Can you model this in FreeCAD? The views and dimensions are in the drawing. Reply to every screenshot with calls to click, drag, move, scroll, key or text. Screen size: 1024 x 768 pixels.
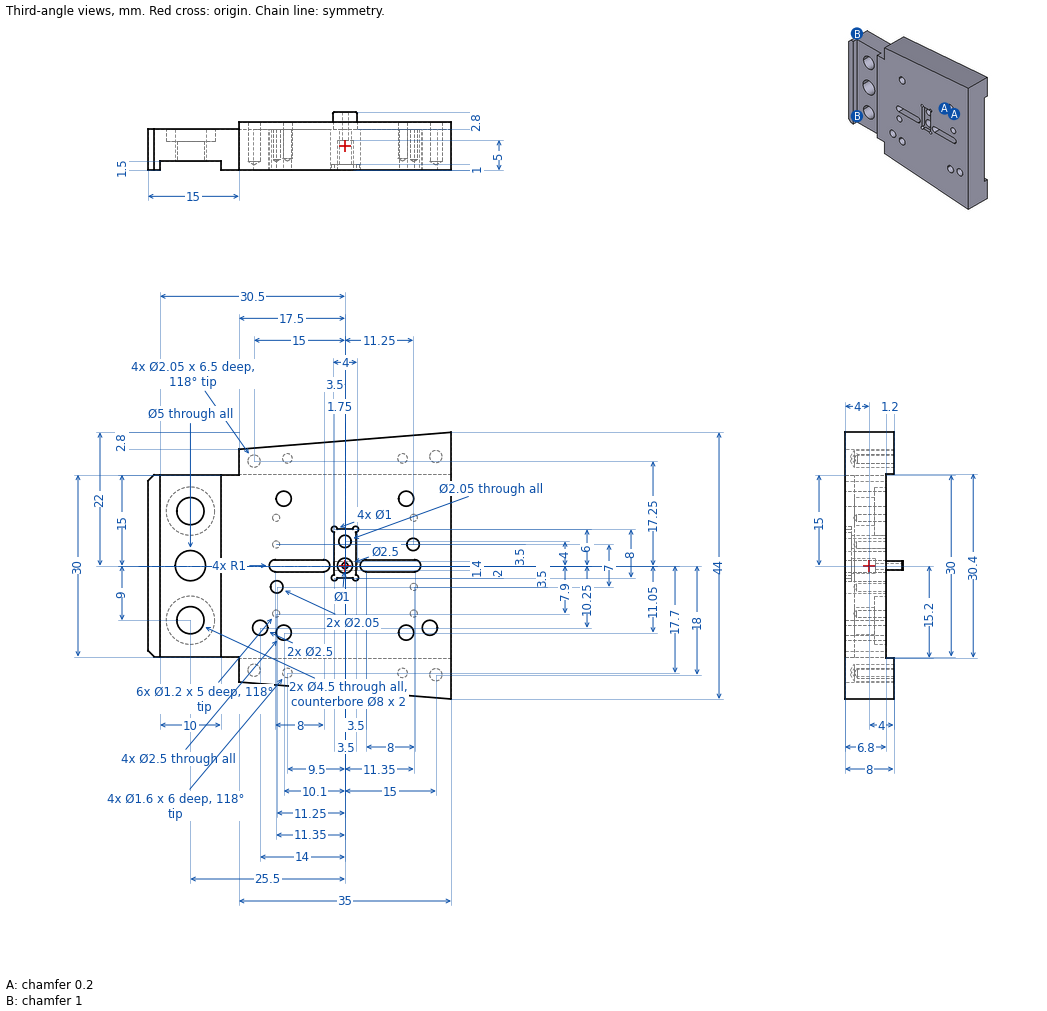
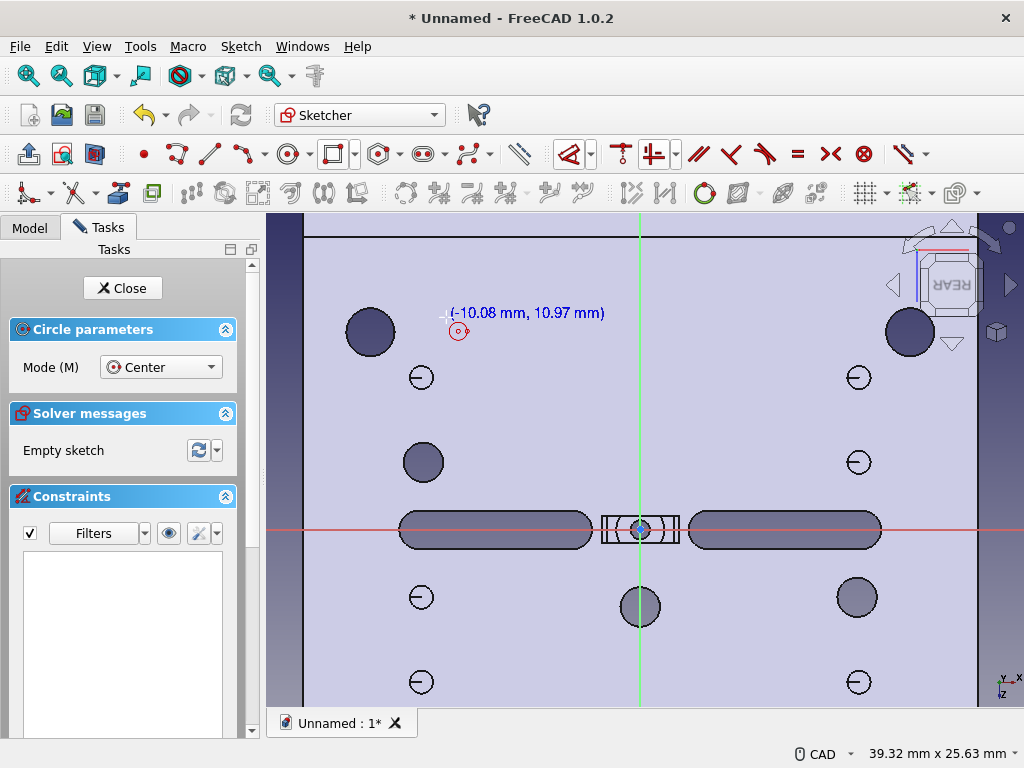
click(446, 317)
move(463, 300)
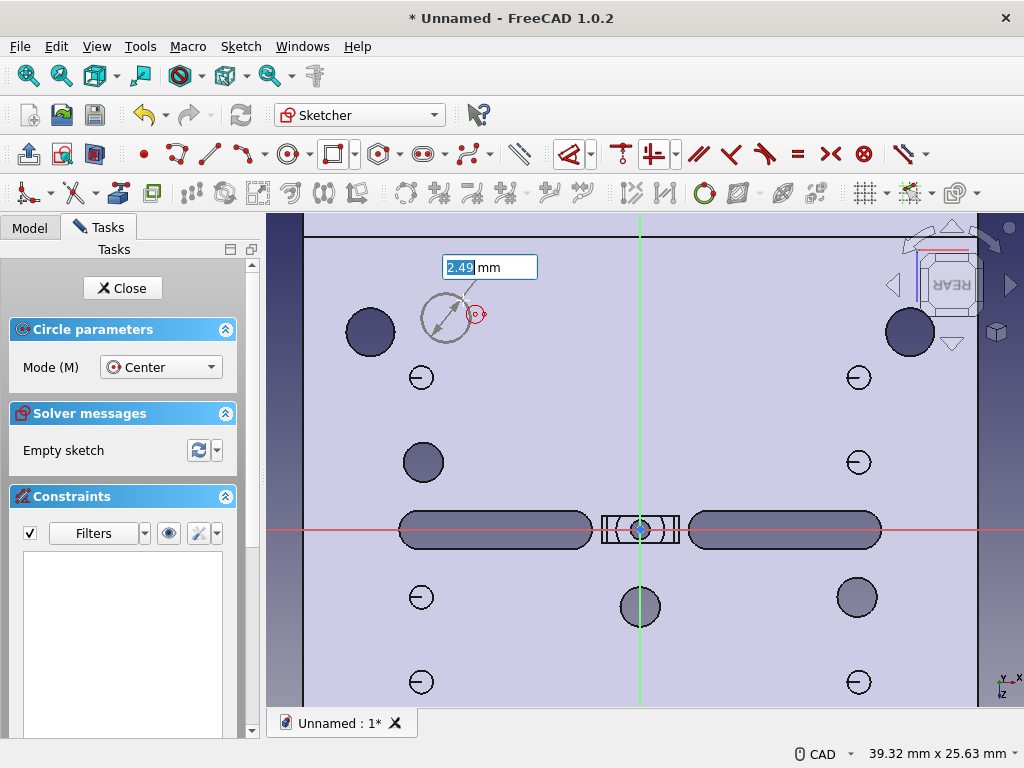
text(2.5)
key(Return)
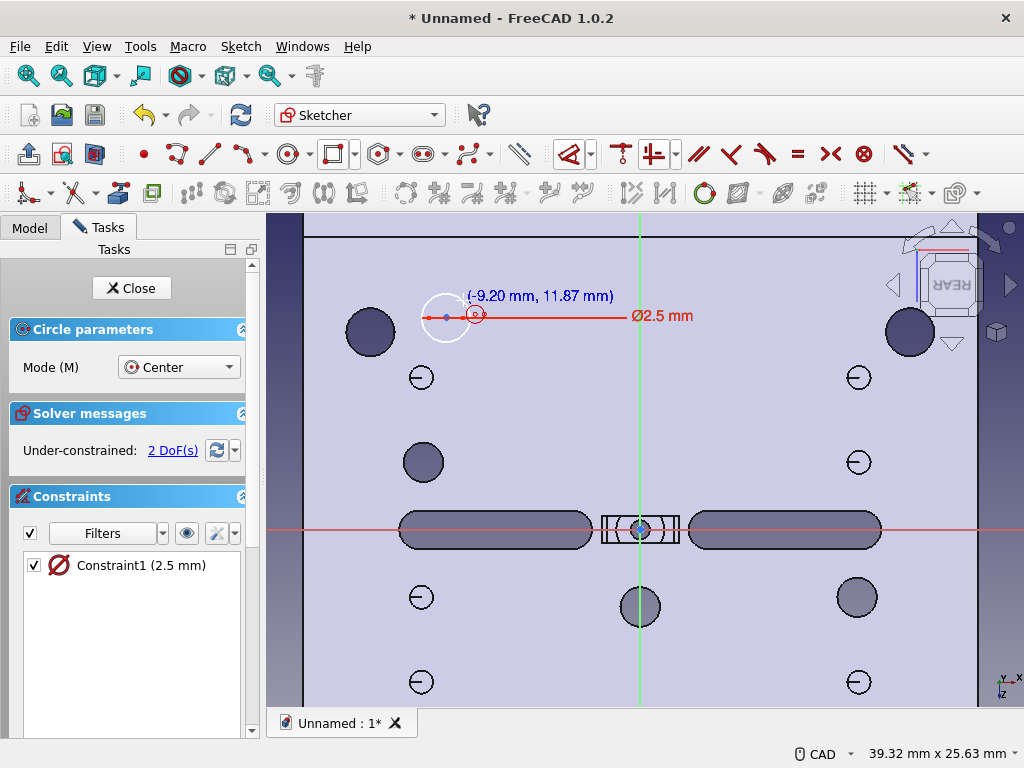
click(835, 317)
move(852, 300)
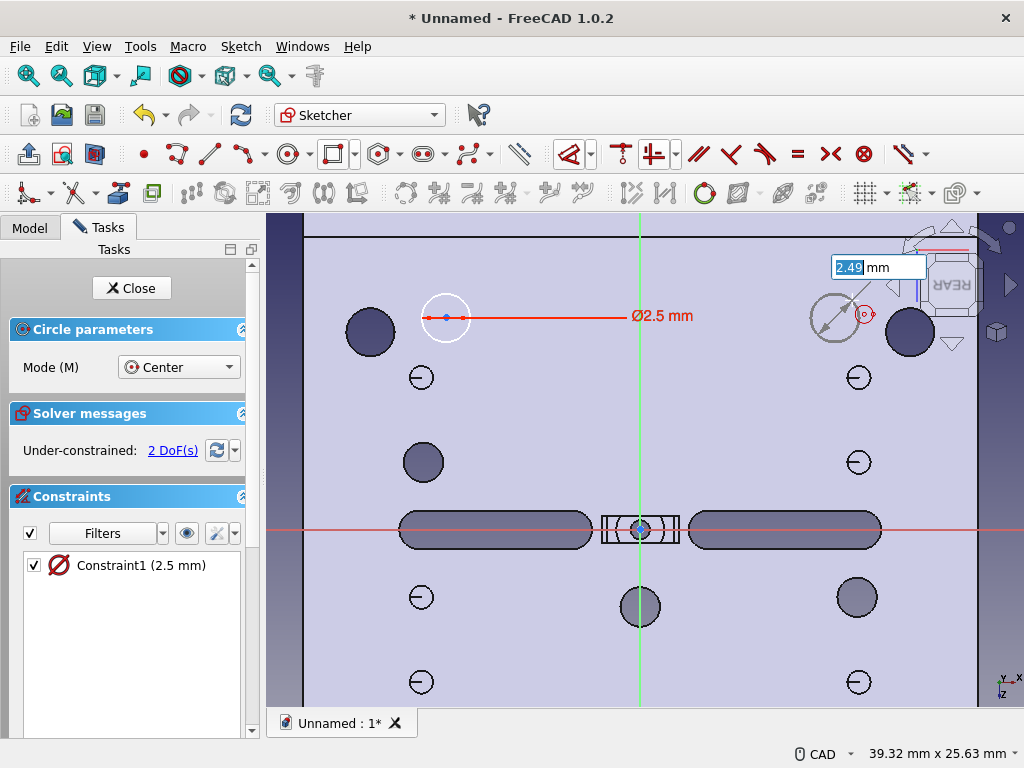
text(2.5)
key(Return)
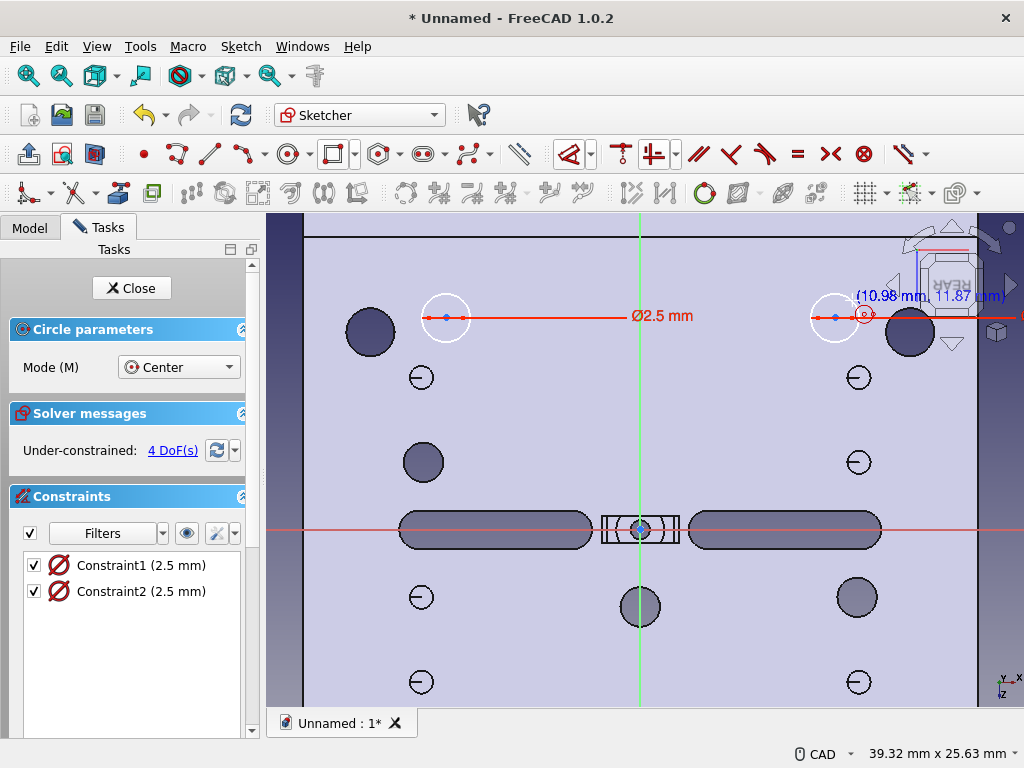
scroll(447, 318, down, 2)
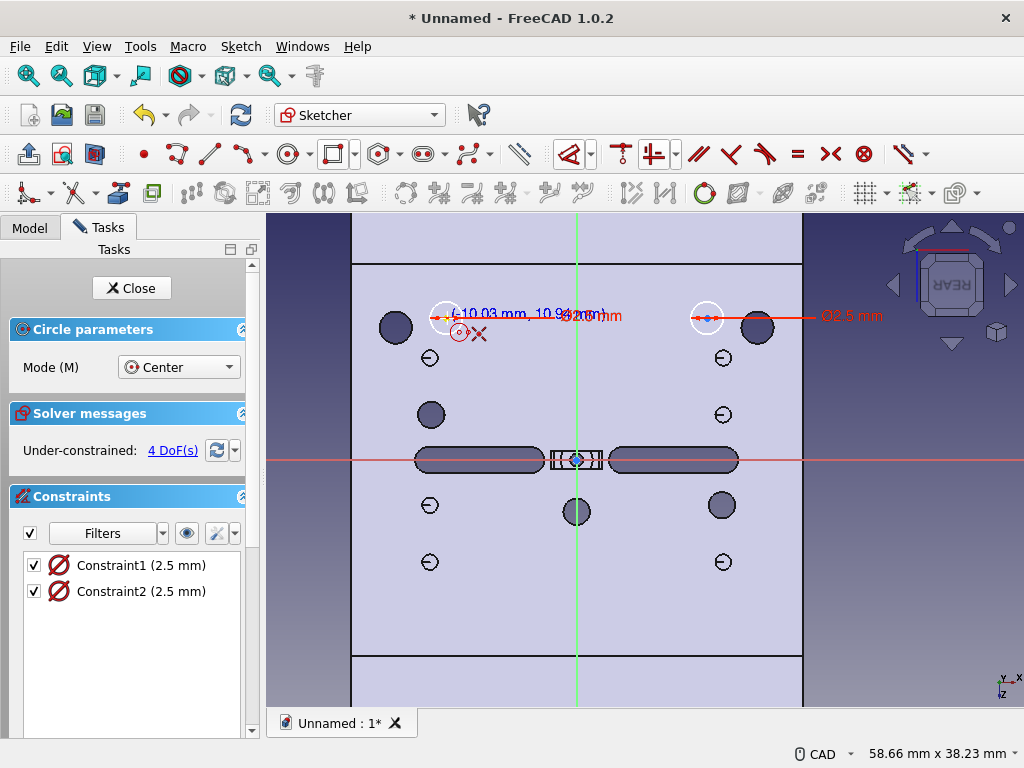
scroll(446, 603, up, 2)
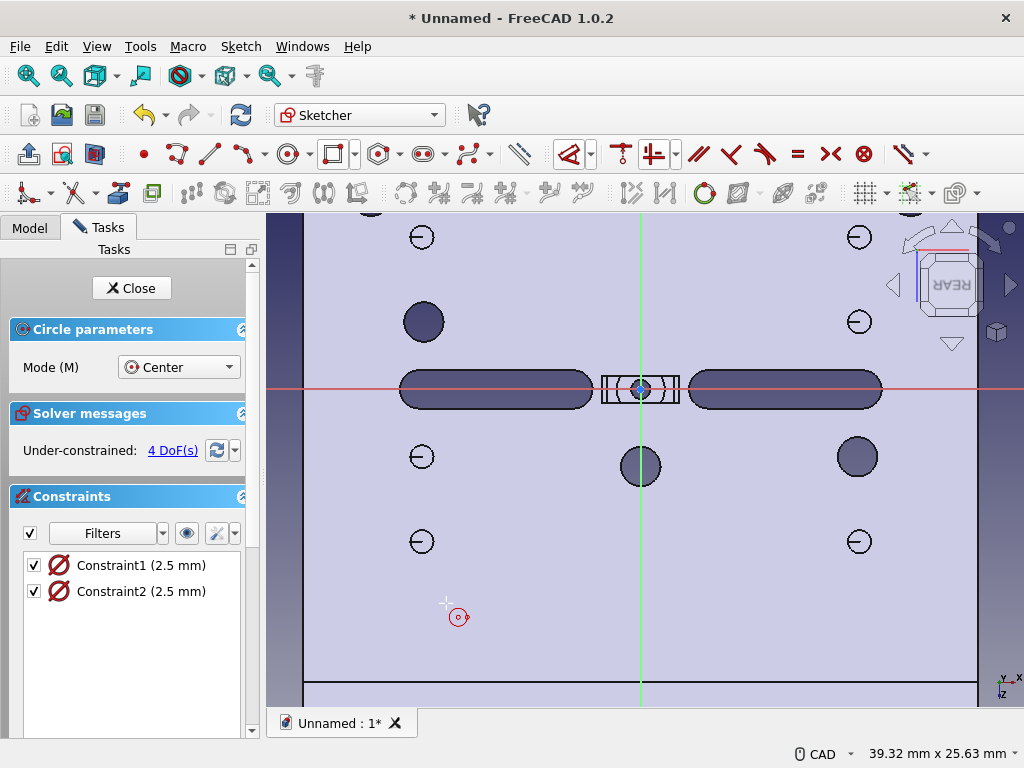
click(446, 602)
move(463, 585)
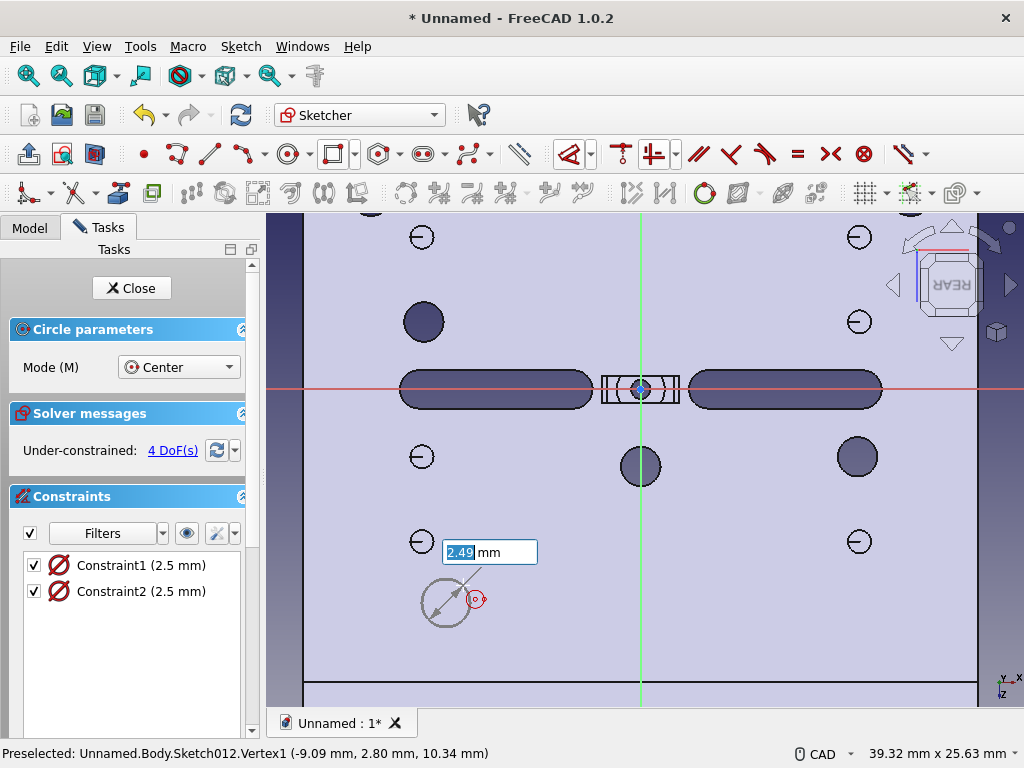
text(2.5)
key(Return)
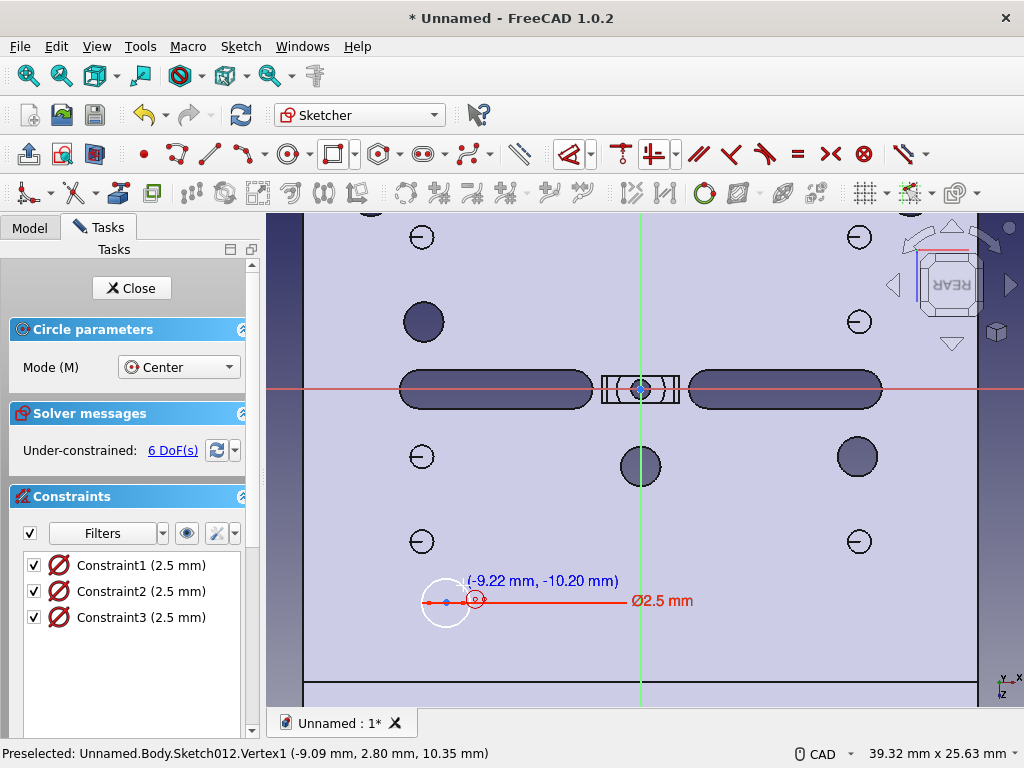
click(835, 602)
move(852, 585)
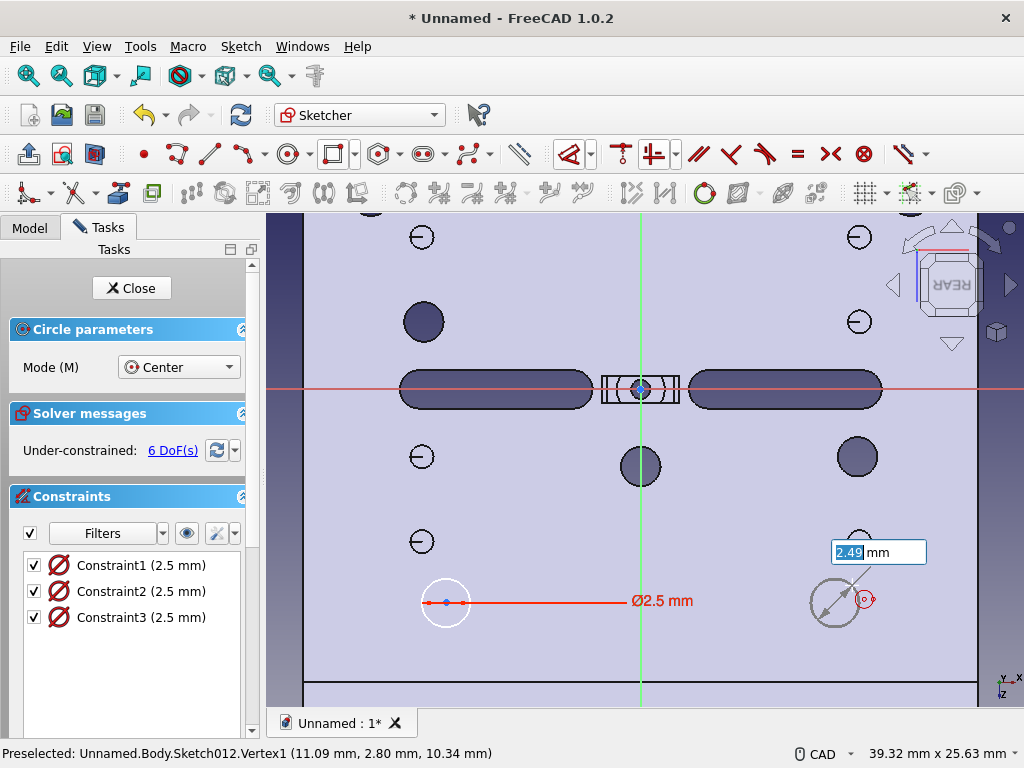
text(2.5)
key(Return)
key(Escape)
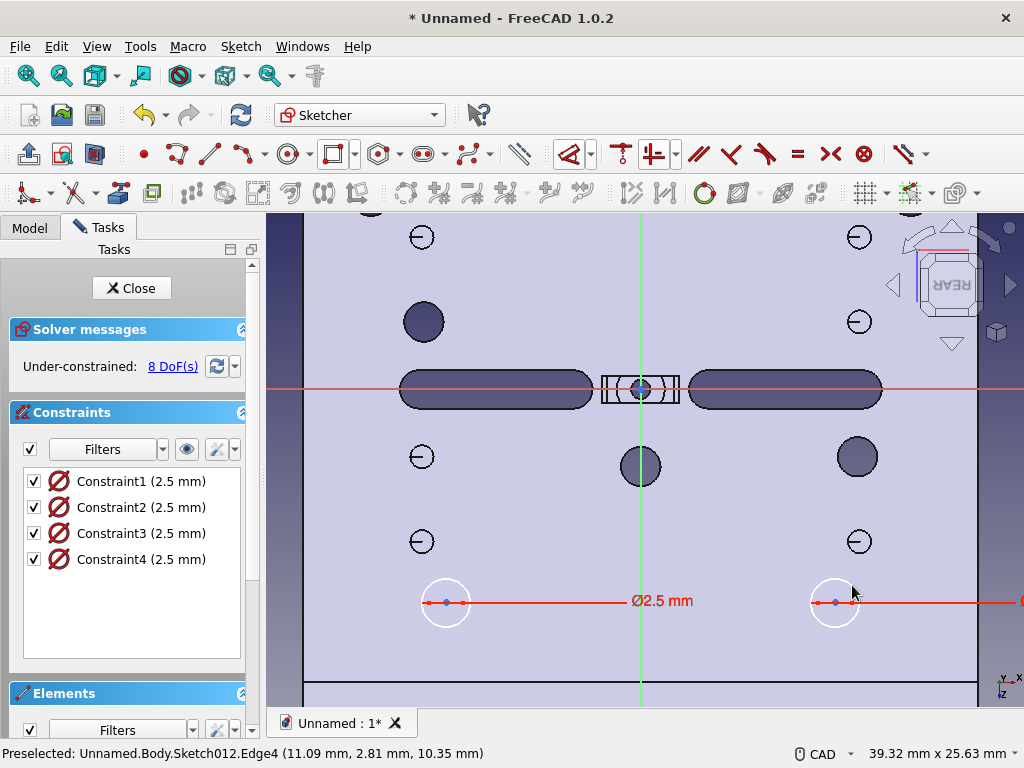
scroll(446, 604, down, 2)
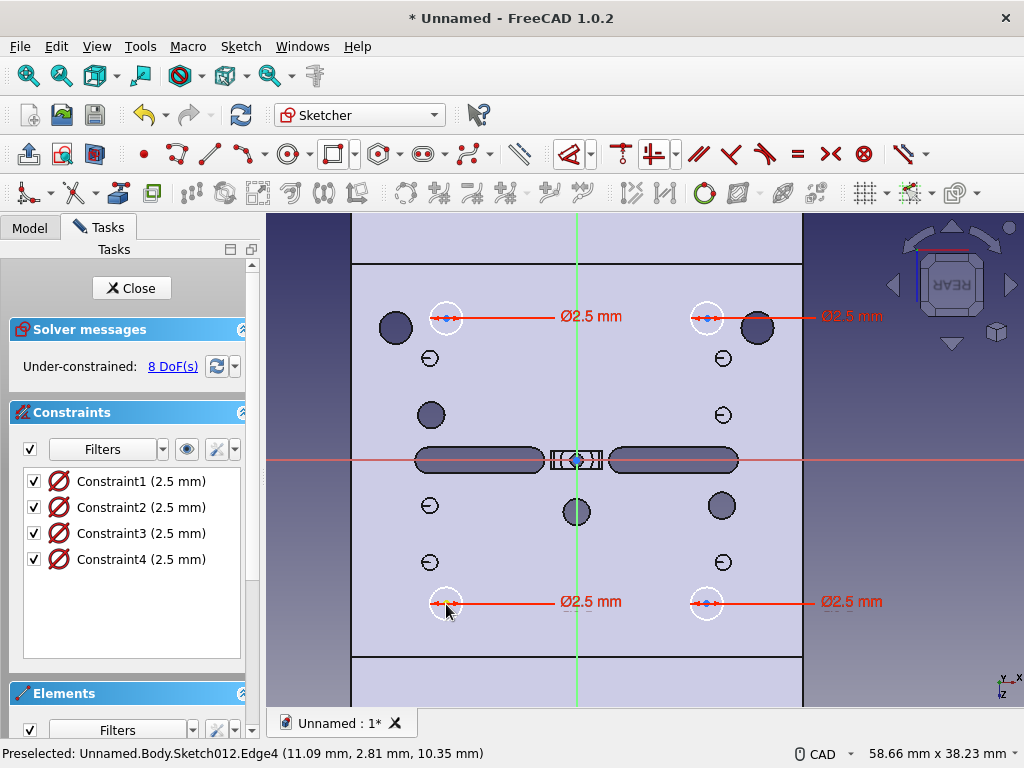
click(446, 318)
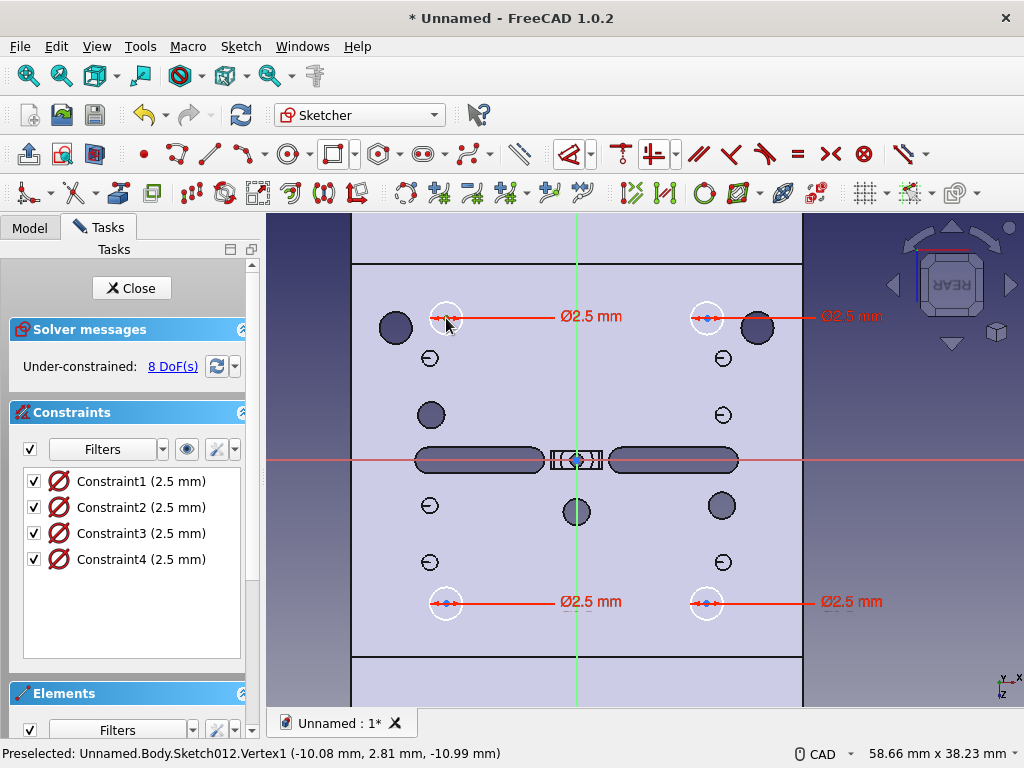
click(707, 318)